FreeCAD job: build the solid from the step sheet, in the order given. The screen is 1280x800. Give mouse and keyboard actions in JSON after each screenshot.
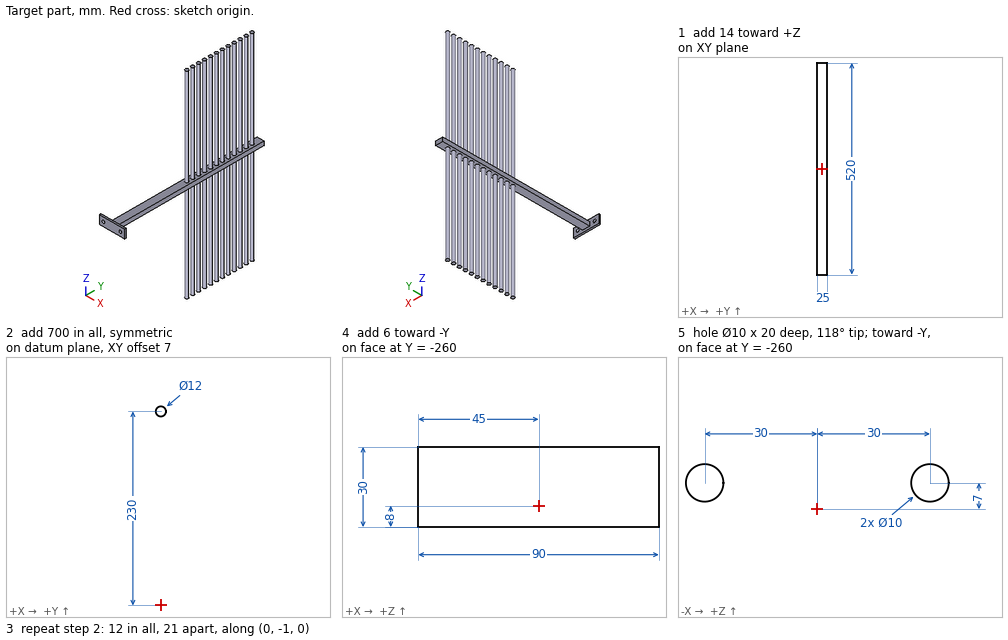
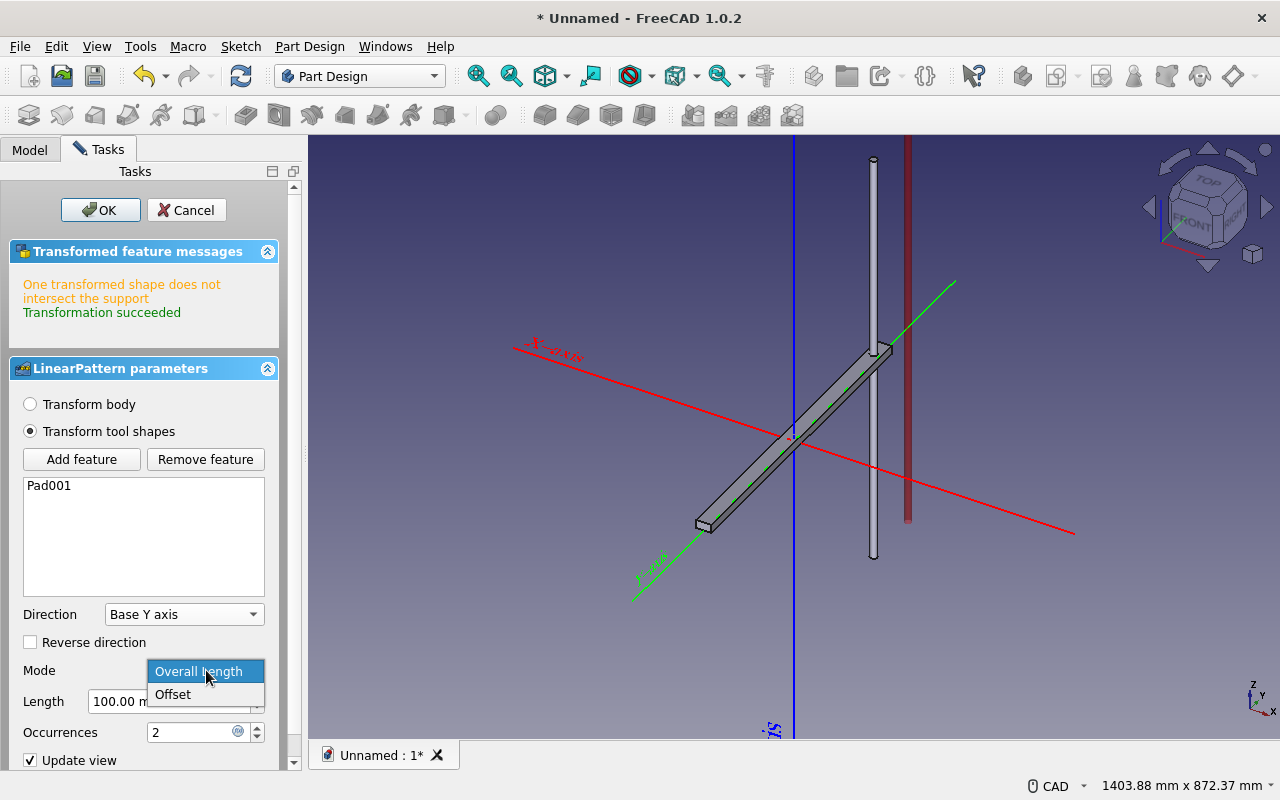
{"action": "left_click", "coordinate": [204, 694]}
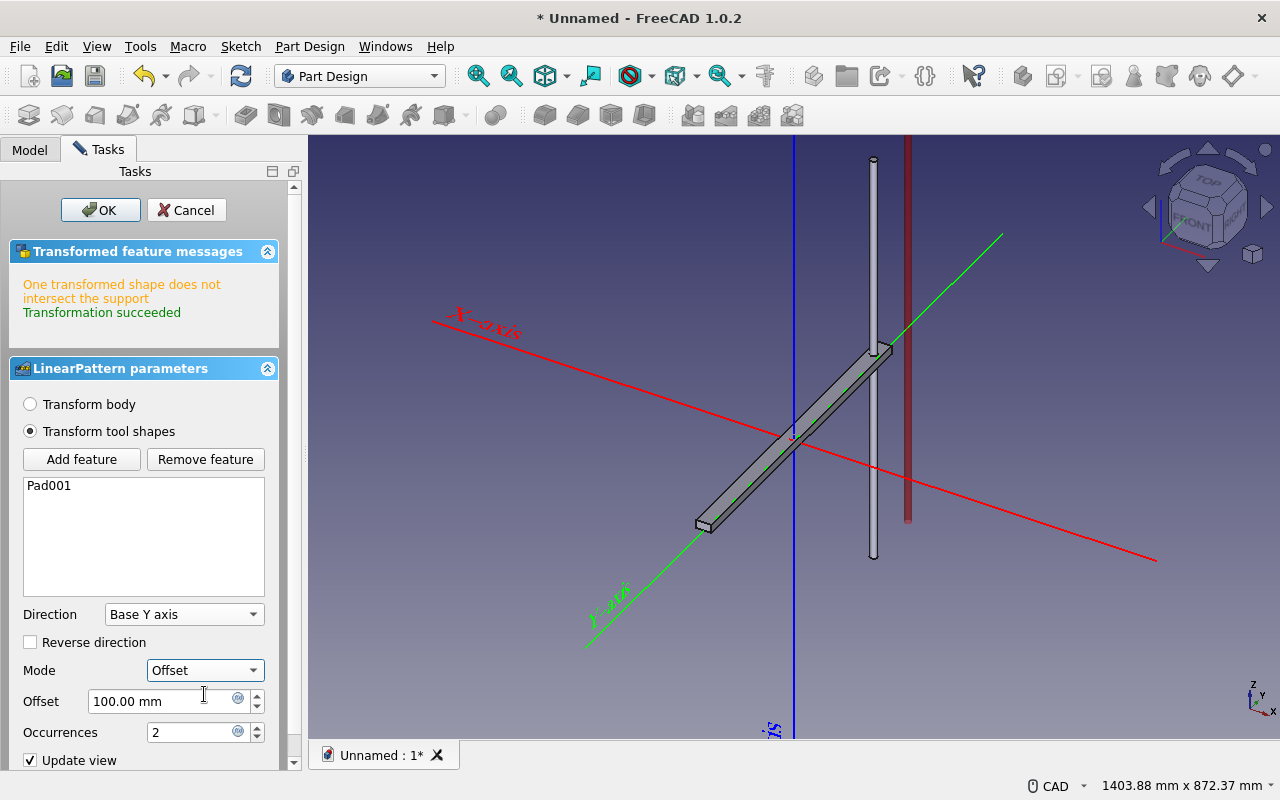
{"action": "triple_click", "coordinate": [170, 702]}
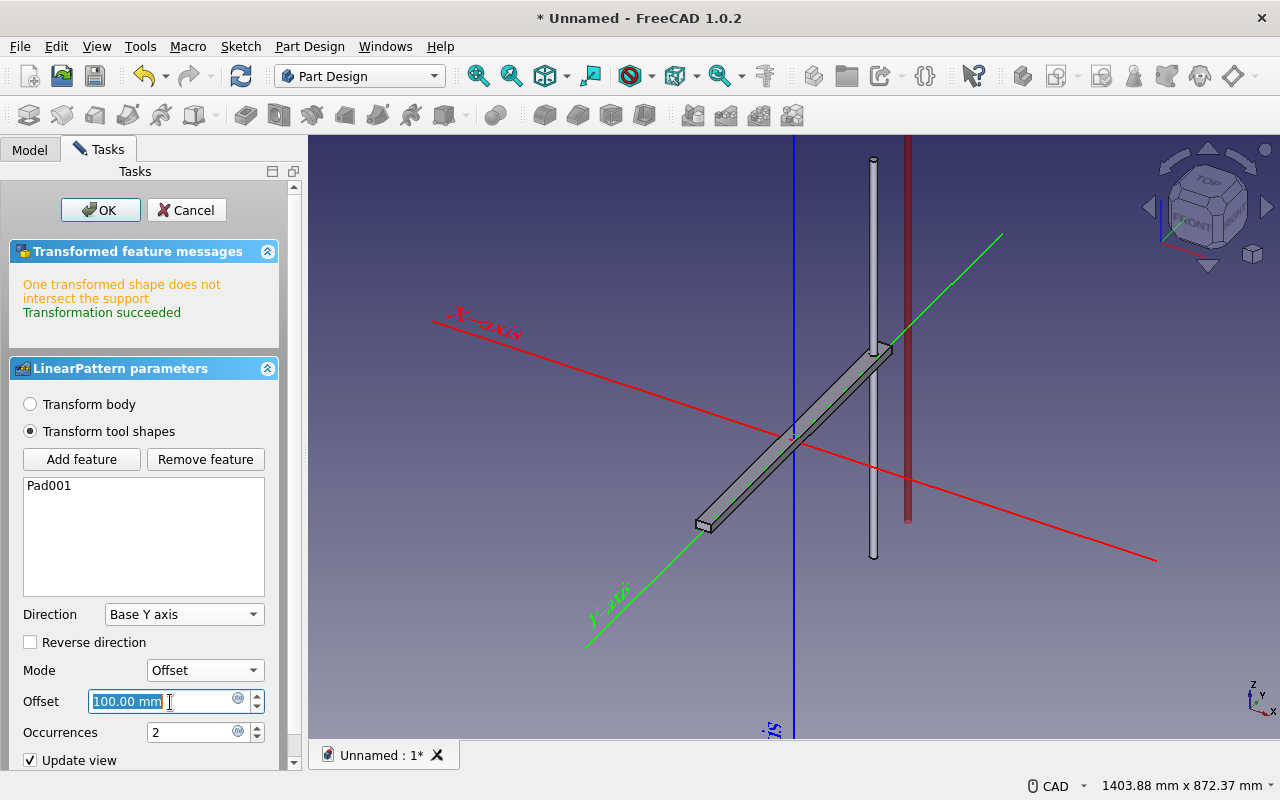
{"action": "type", "text": "21"}
{"action": "key", "text": "Tab"}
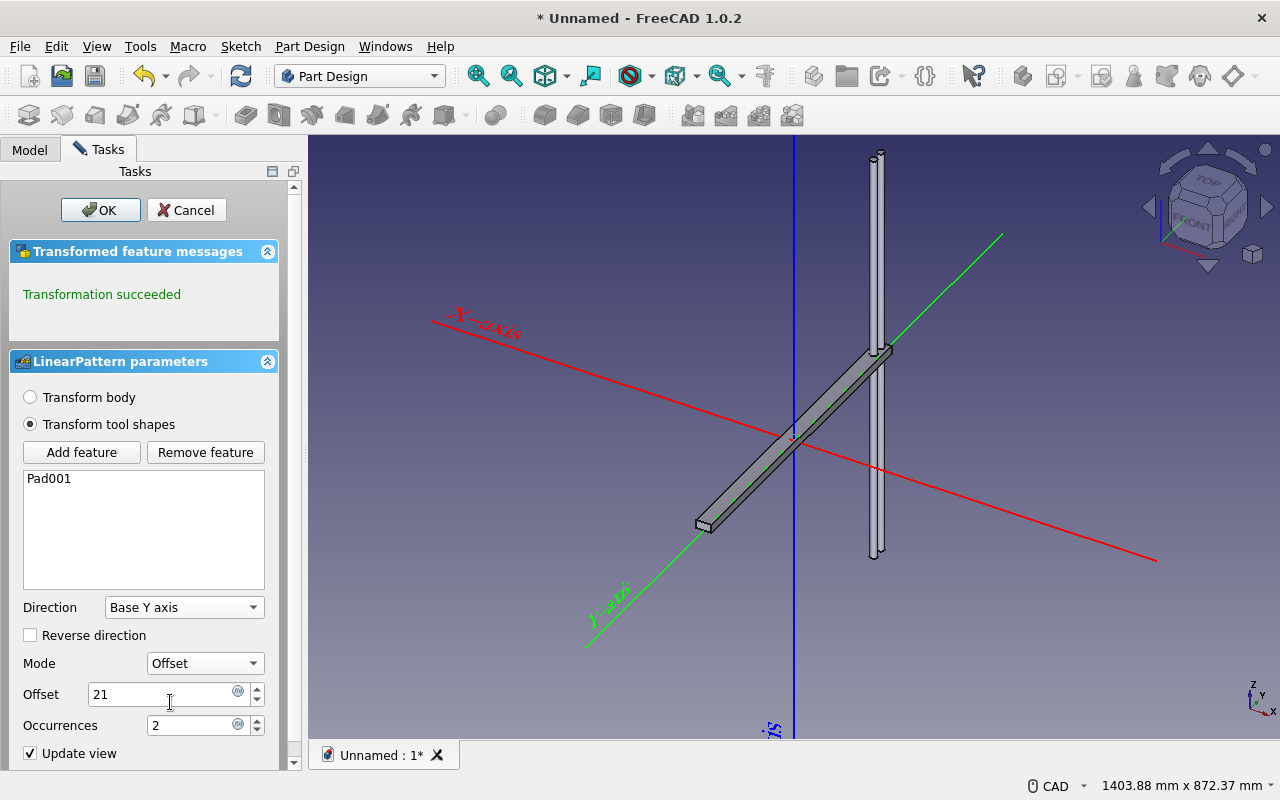
{"action": "triple_click", "coordinate": [199, 726]}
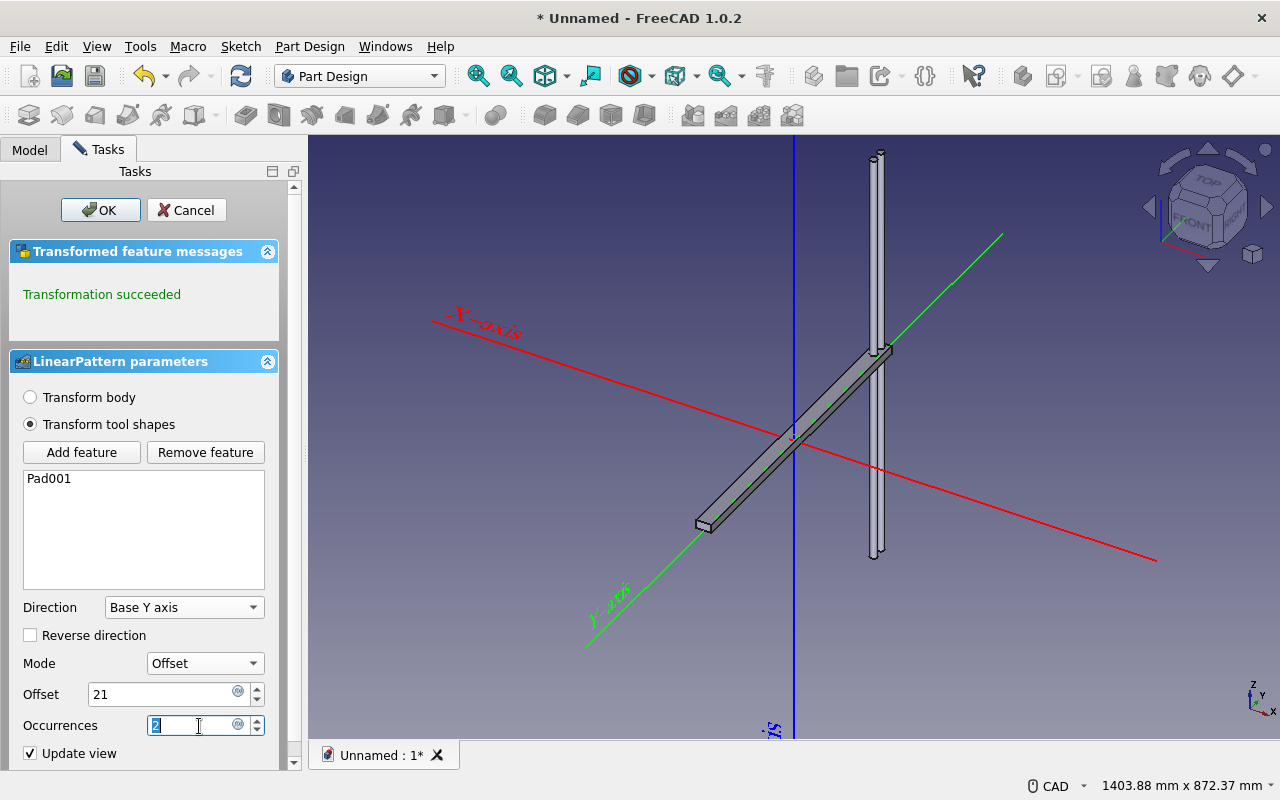
{"action": "type", "text": "12"}
{"action": "key", "text": "Tab"}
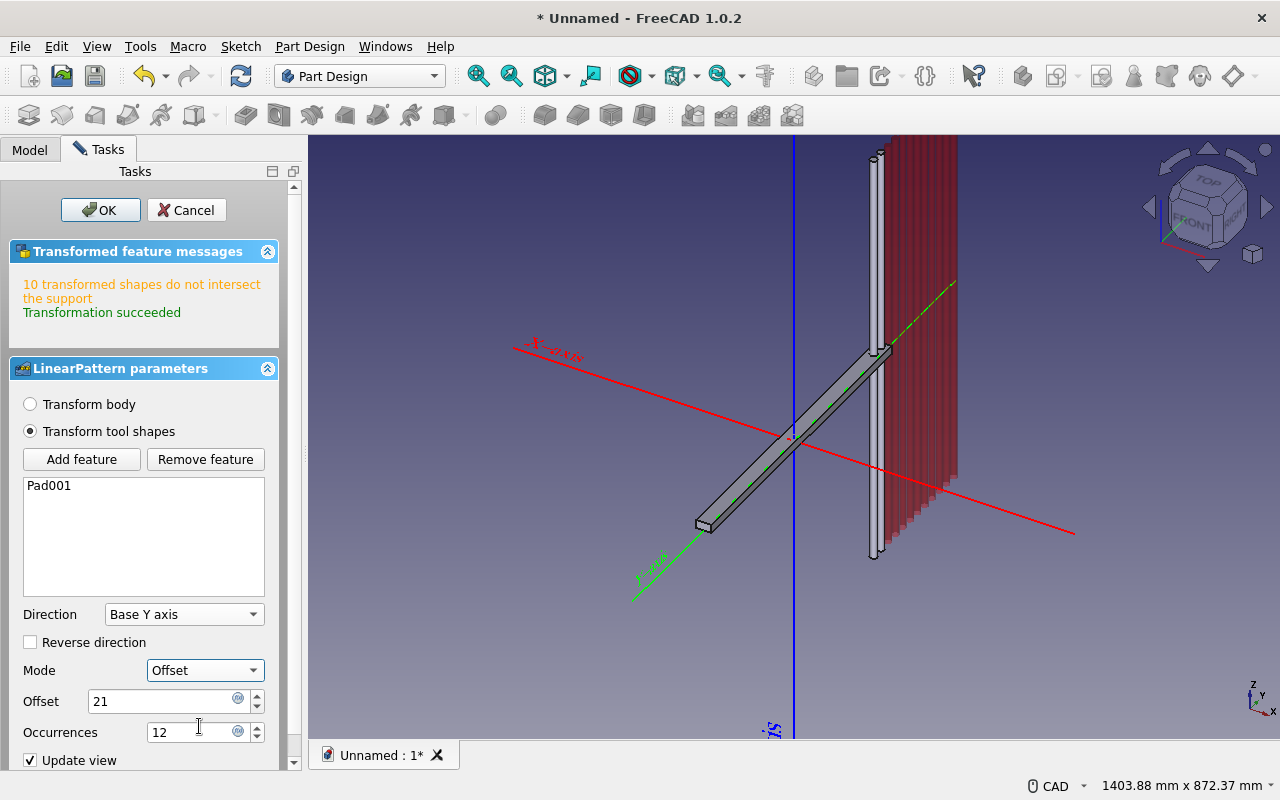
{"action": "left_click", "coordinate": [31, 642]}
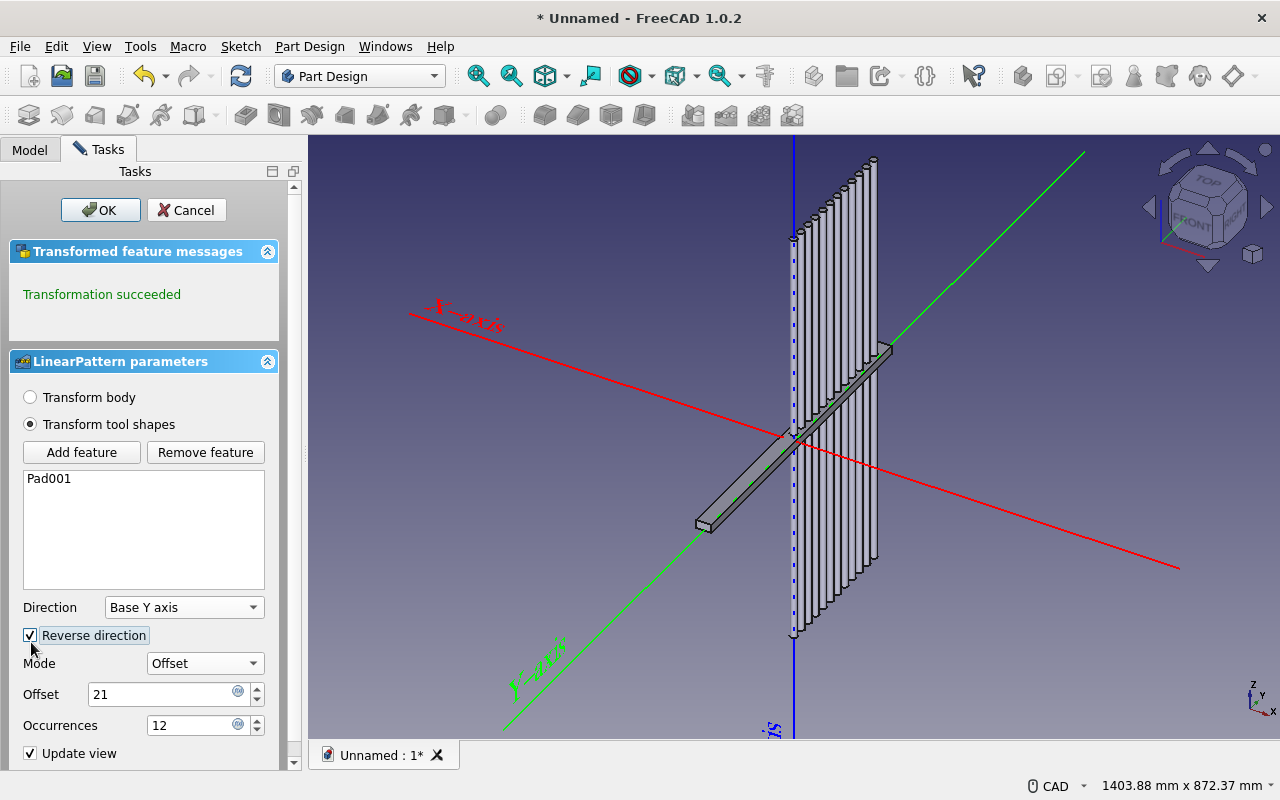
{"action": "left_click", "coordinate": [101, 210]}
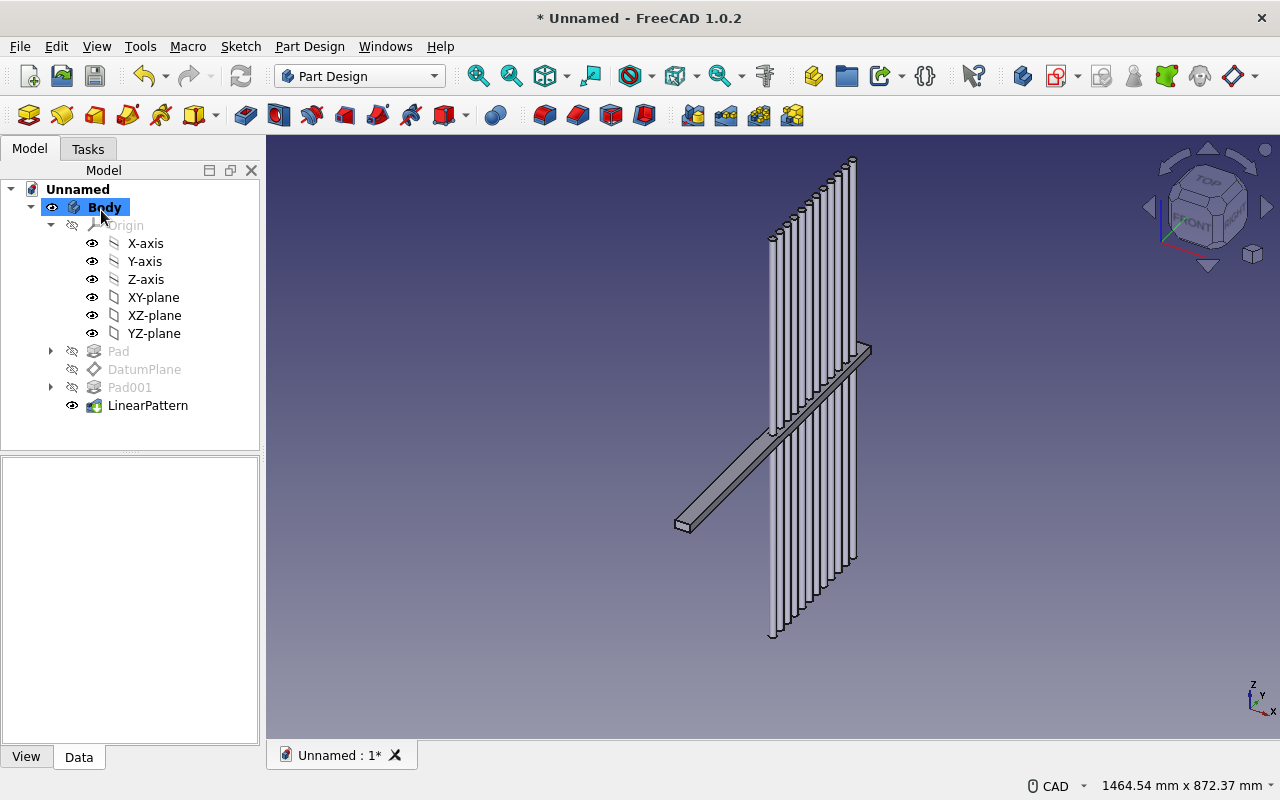
{"action": "scroll", "coordinate": [685, 526], "scroll_direction": "up", "scroll_amount": 5}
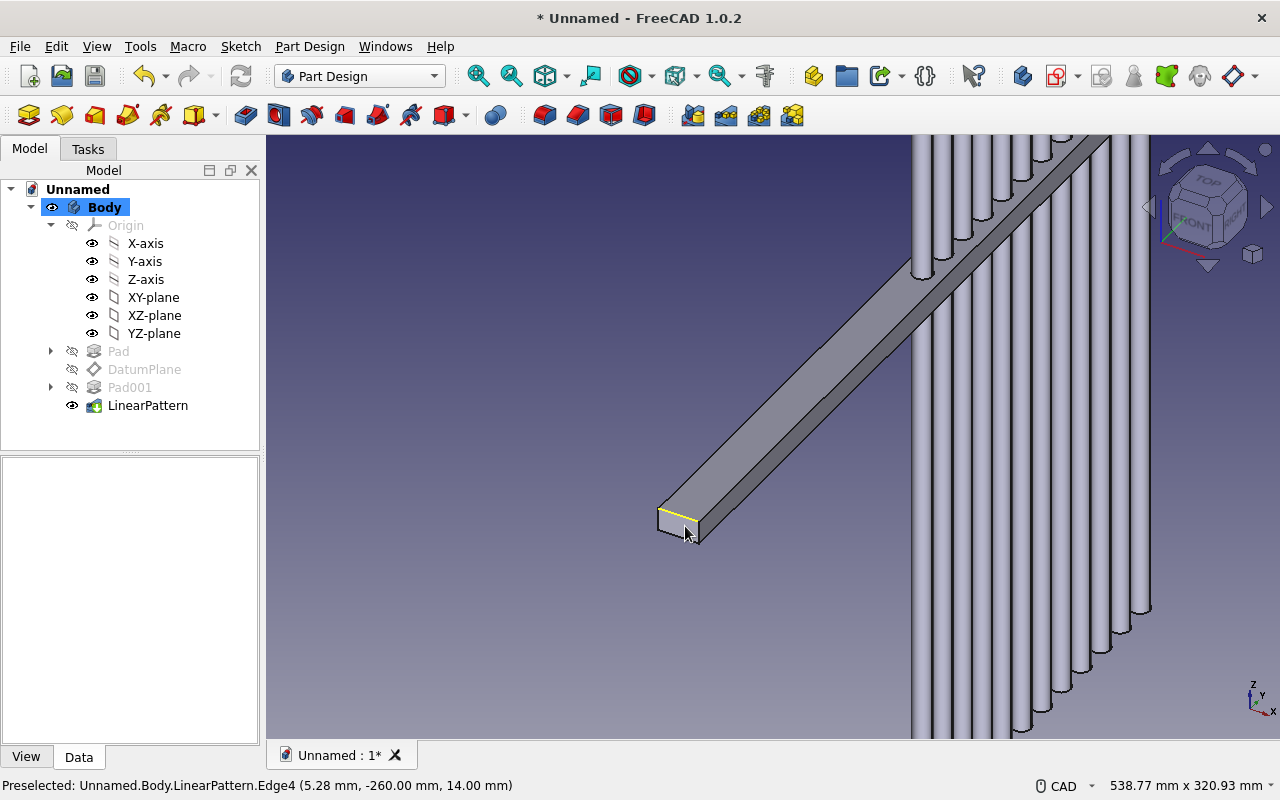
{"action": "left_click", "coordinate": [685, 527]}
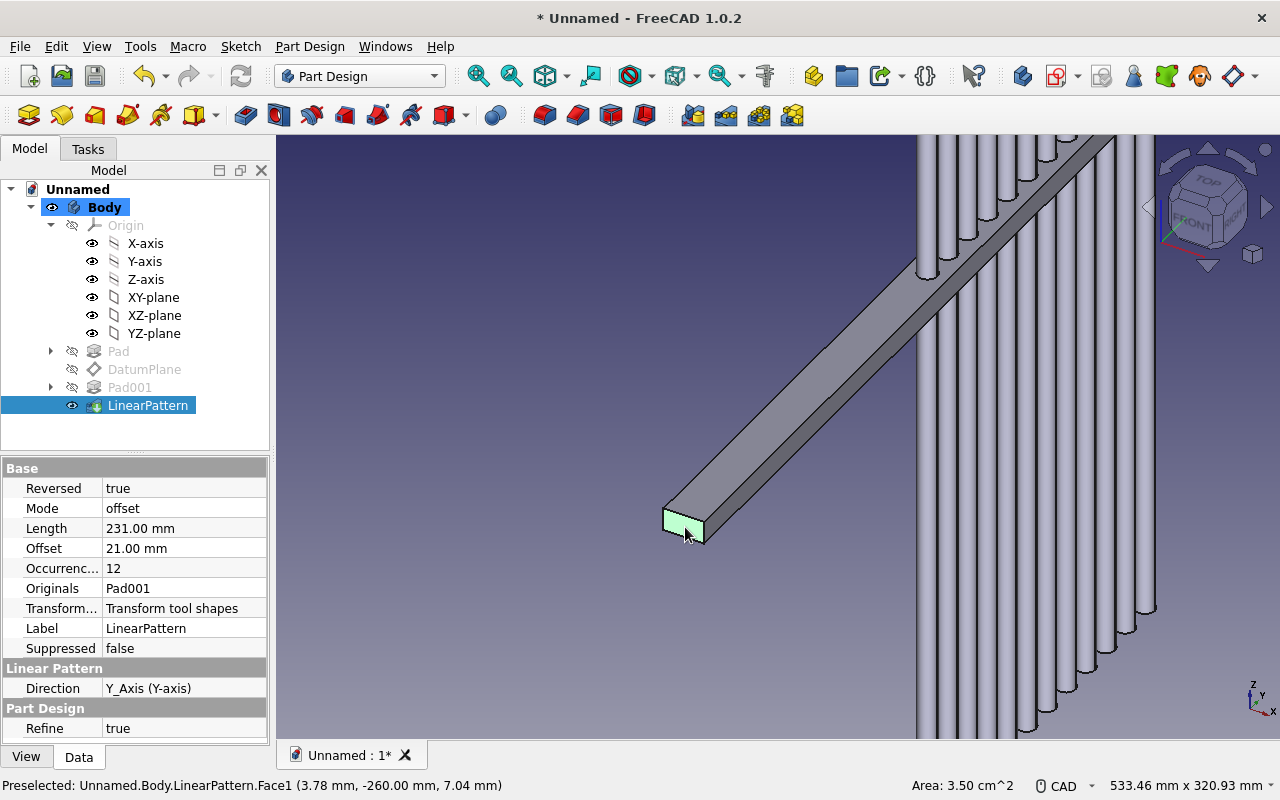
{"action": "left_click", "coordinate": [1056, 76]}